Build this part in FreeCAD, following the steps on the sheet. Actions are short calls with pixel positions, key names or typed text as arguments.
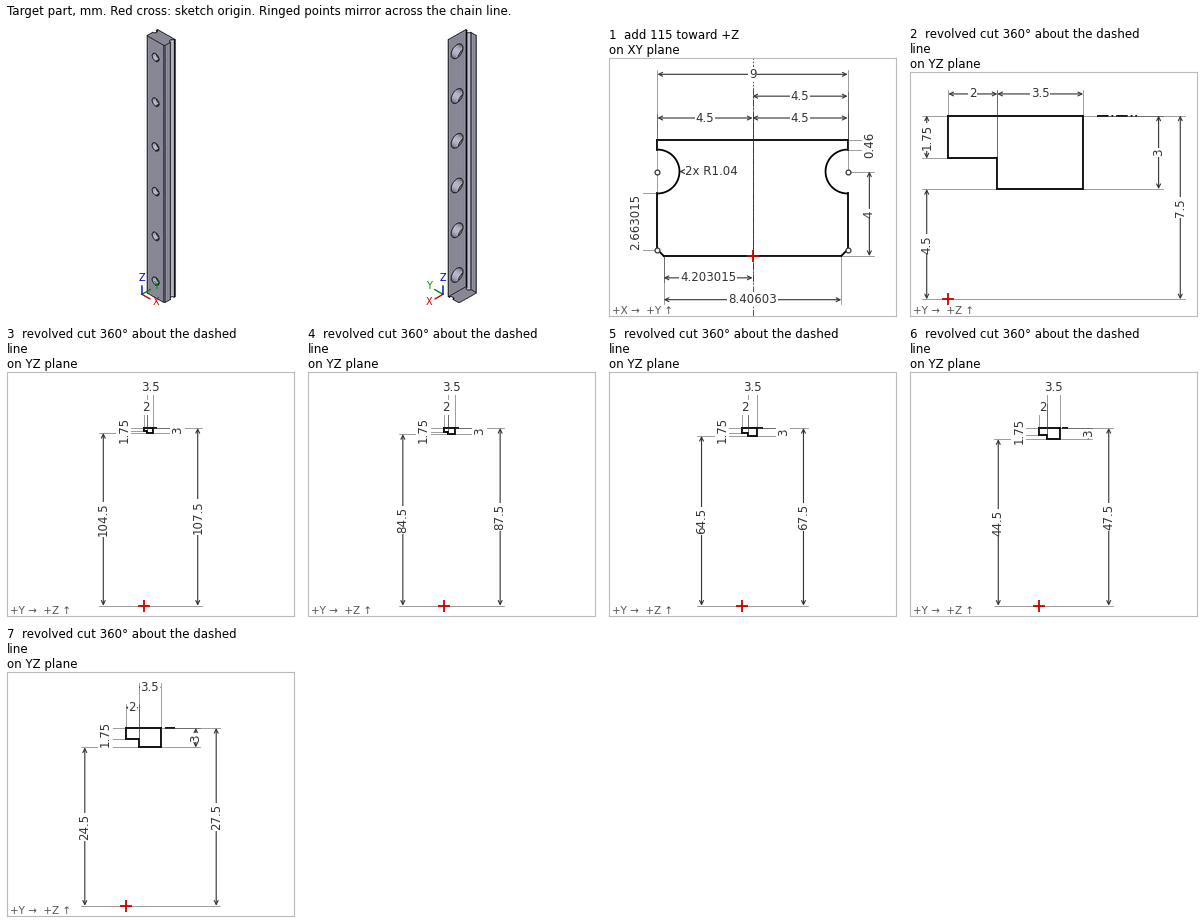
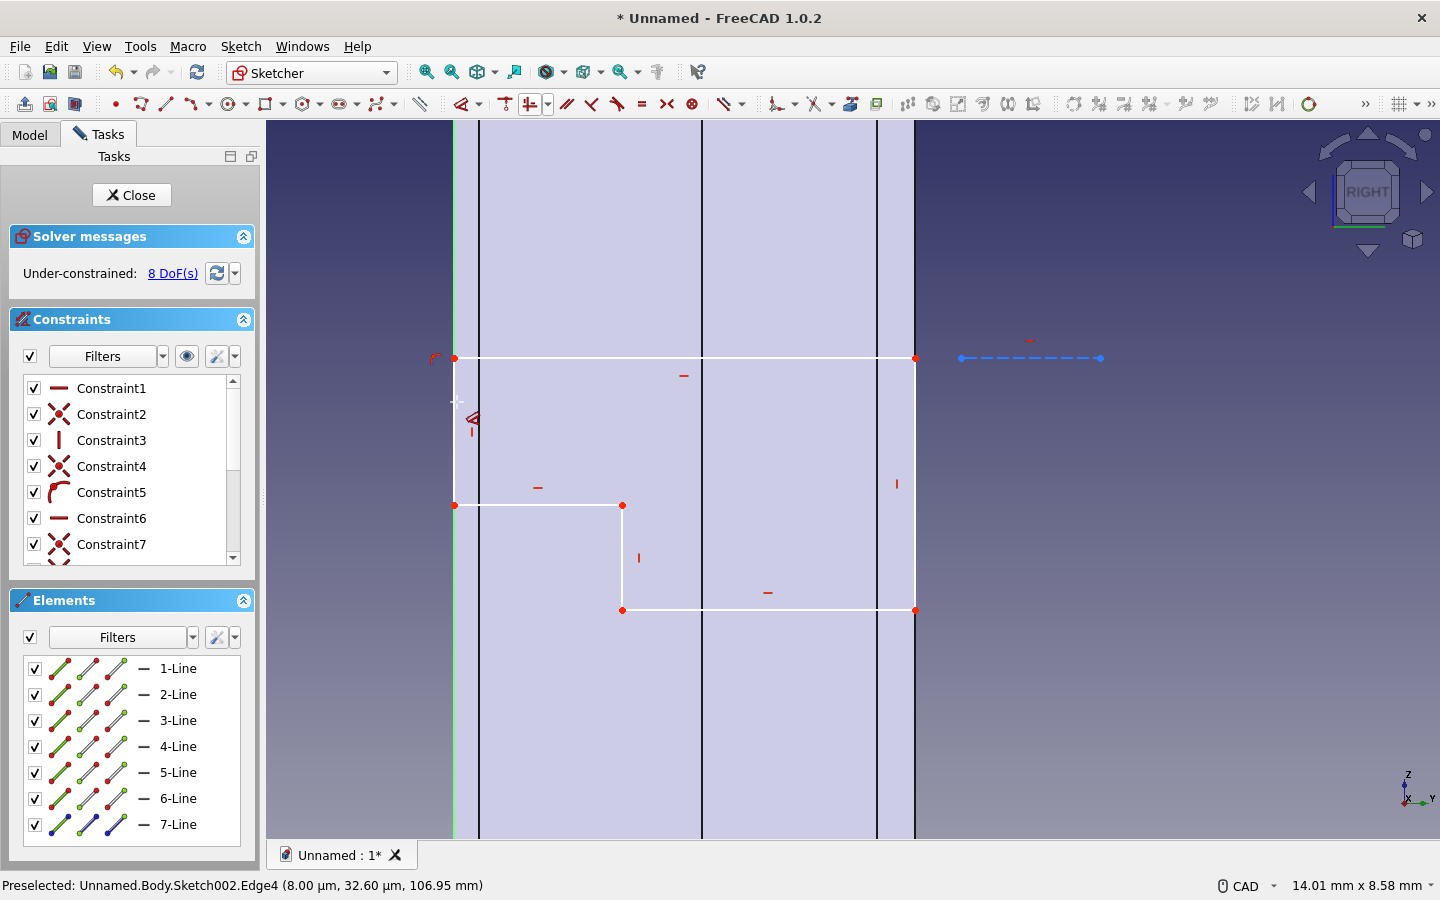
click(915, 534)
click(949, 484)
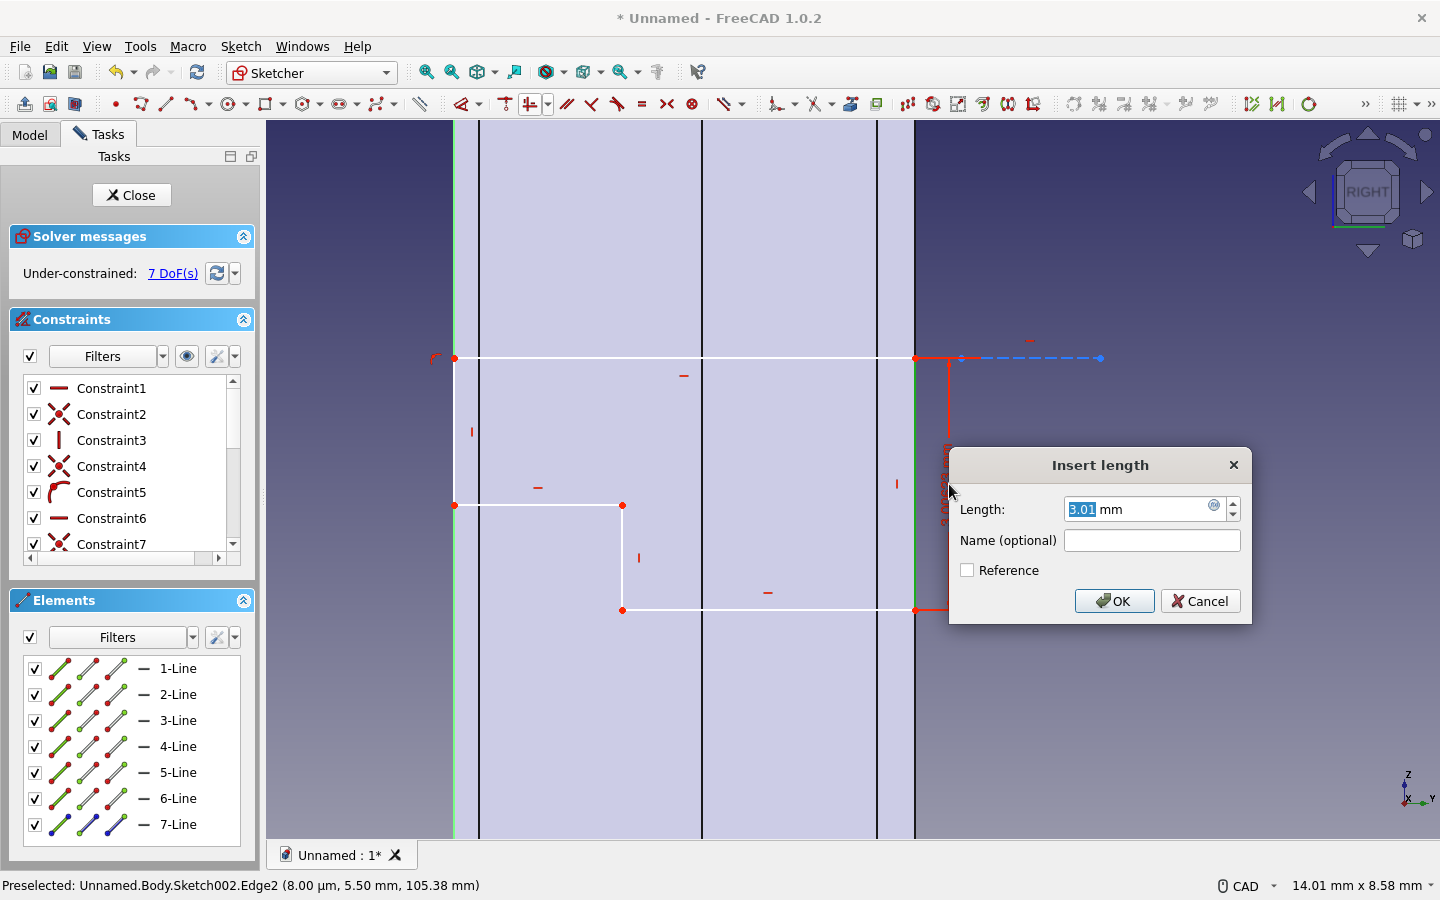
text(3)
key(Return)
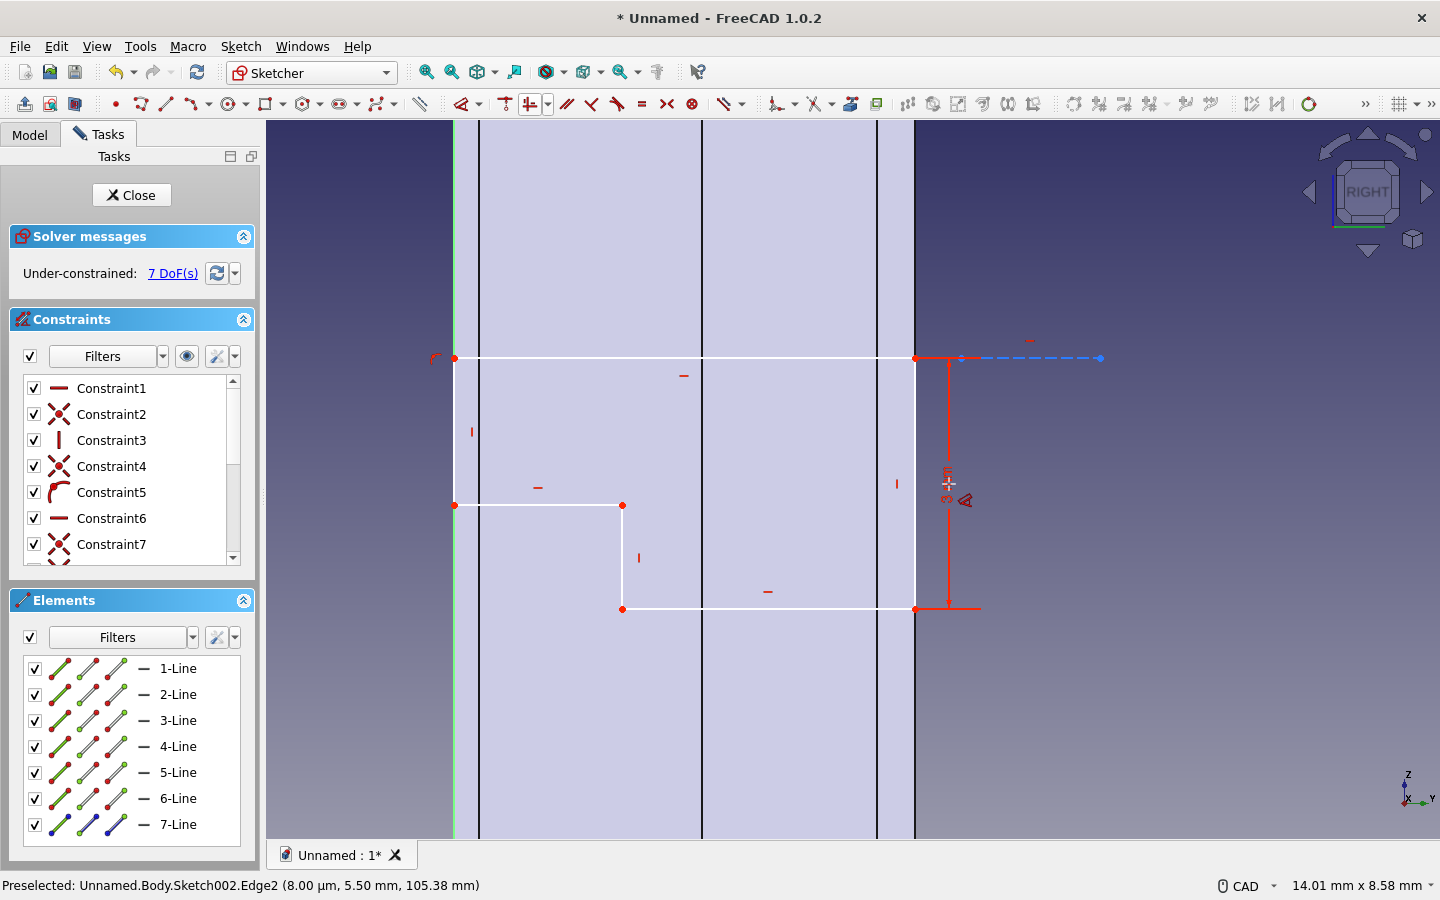
click(504, 505)
click(538, 539)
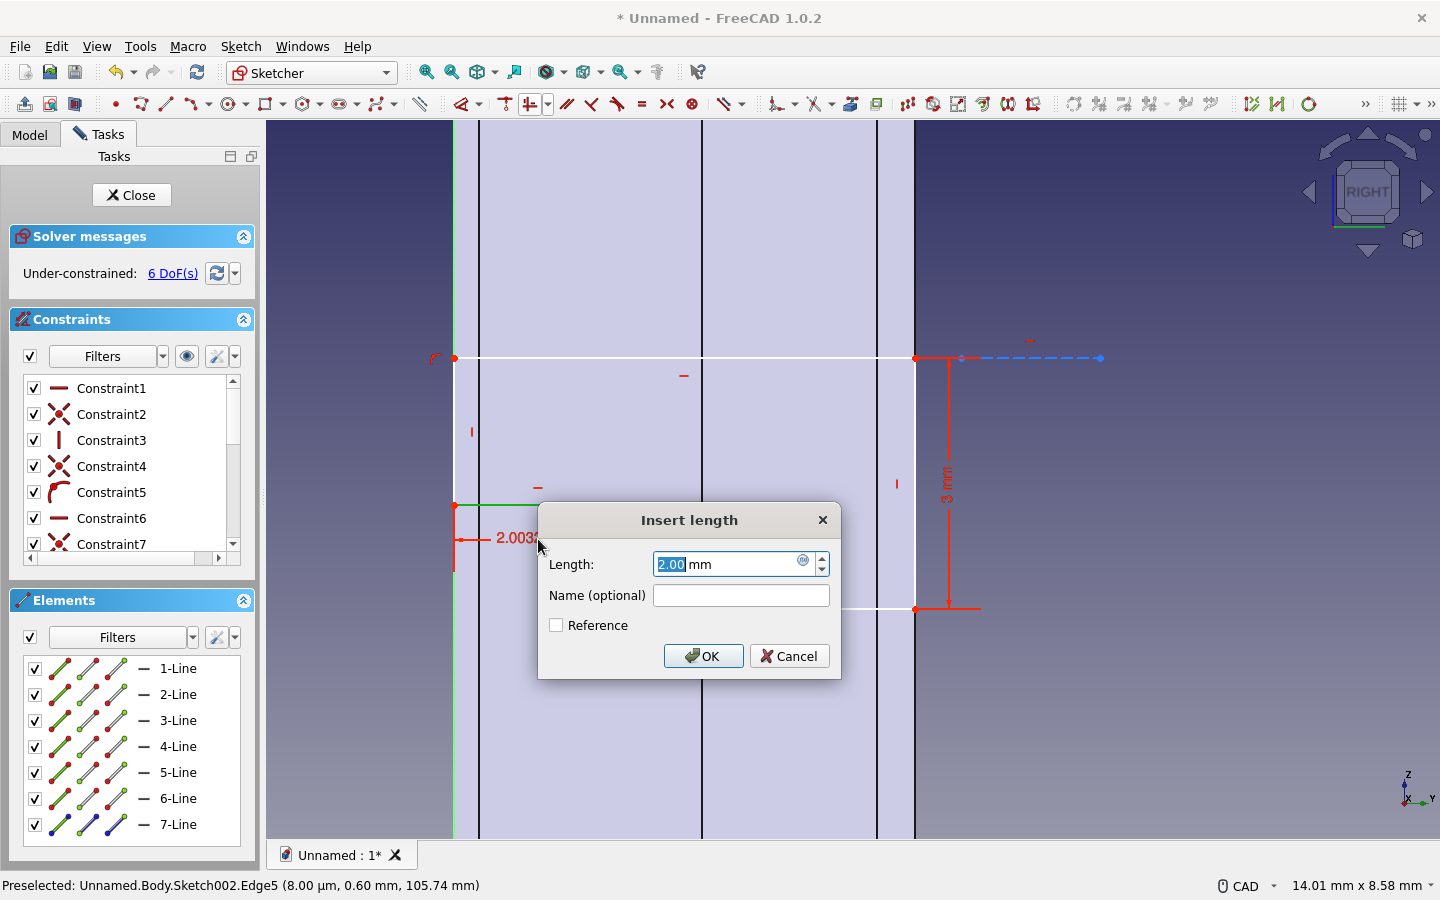
text(2)
key(Return)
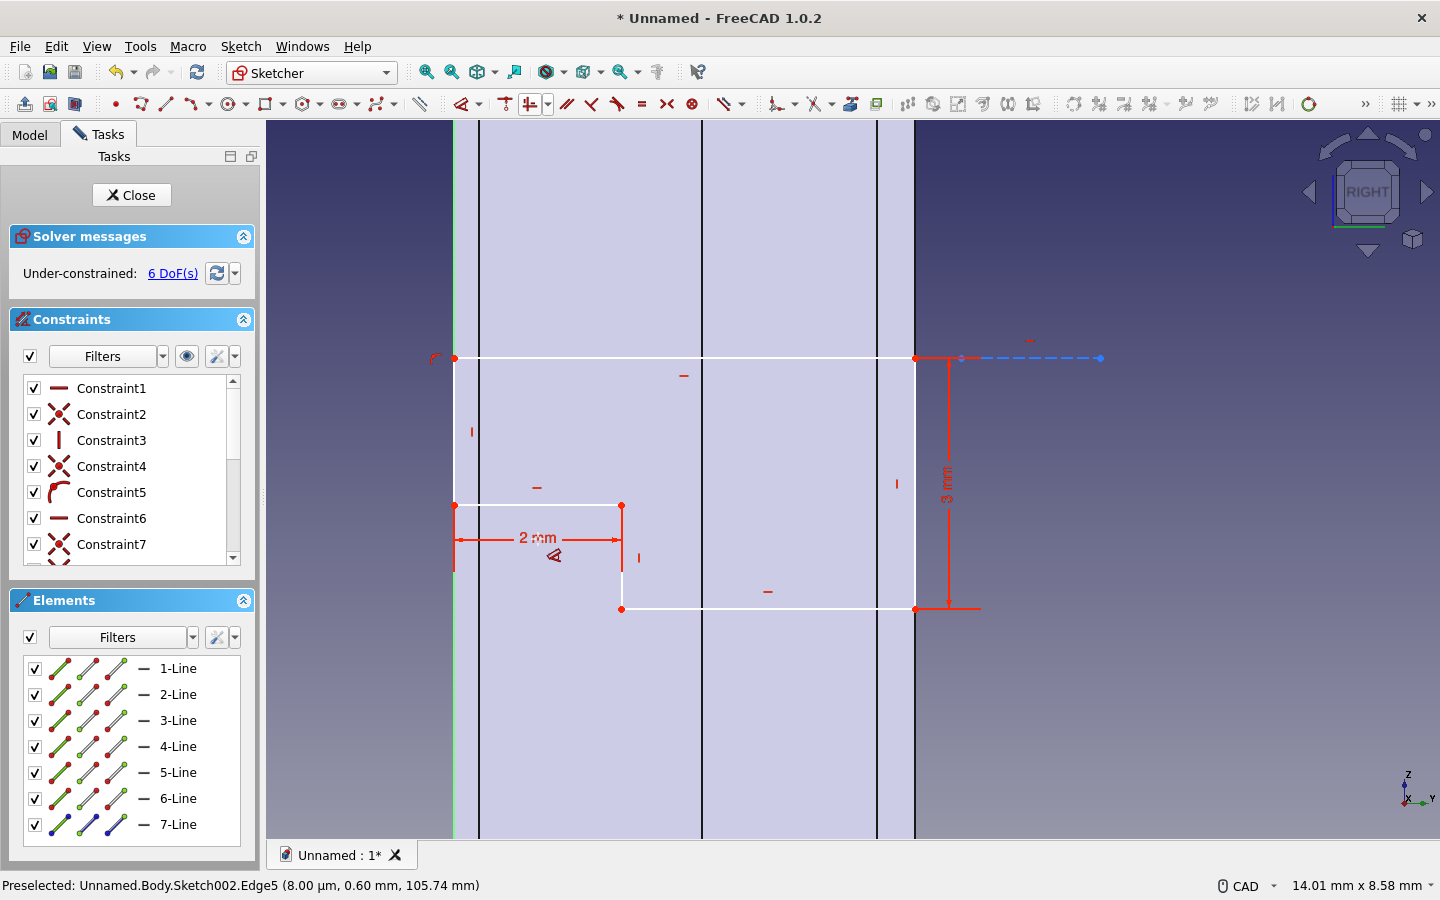
click(710, 609)
click(768, 643)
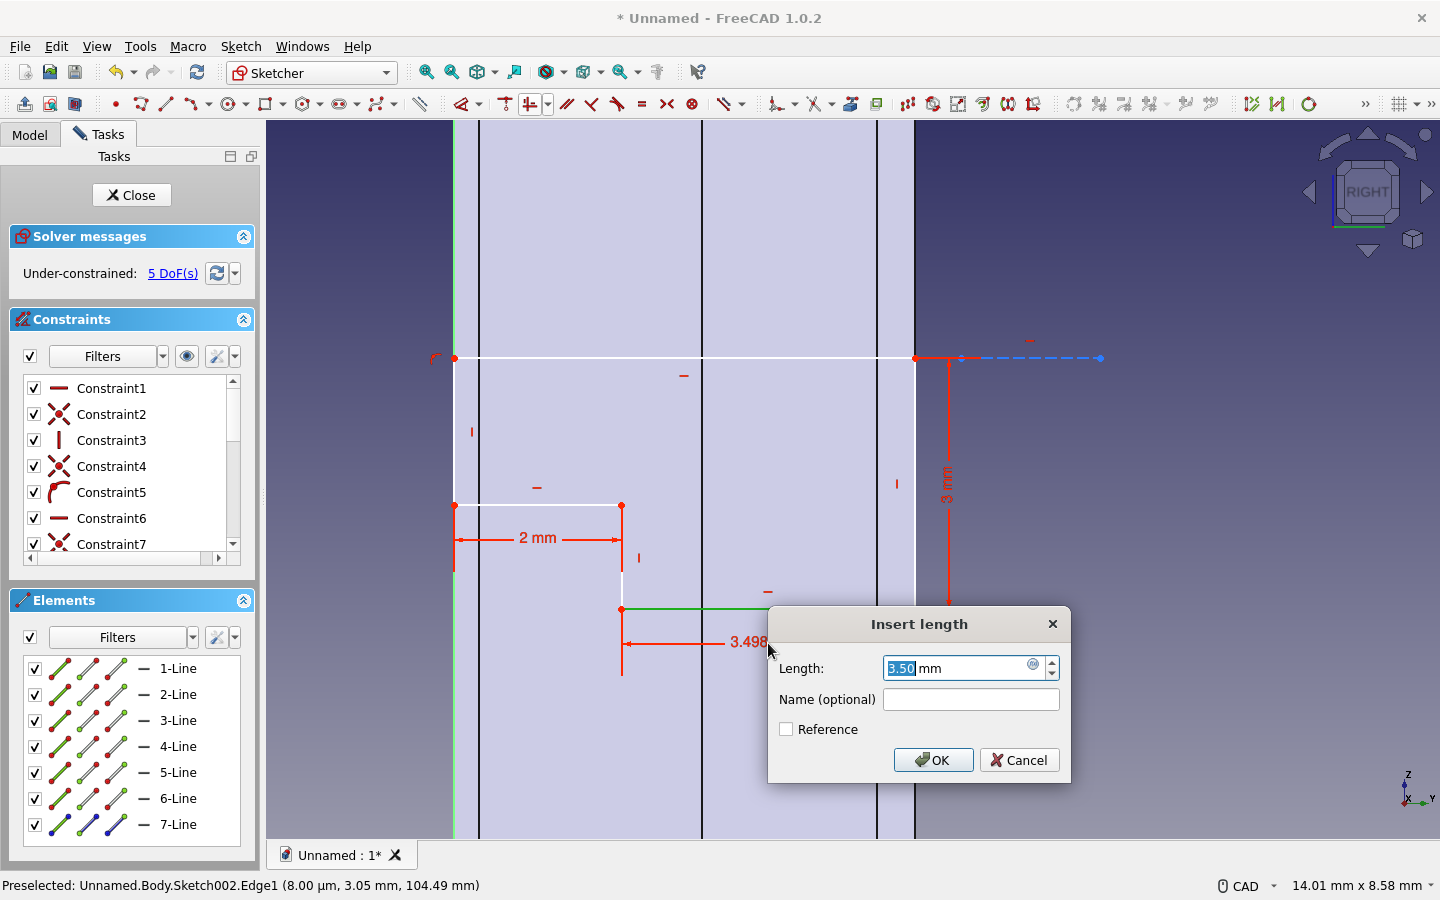
text(3.5)
key(Return)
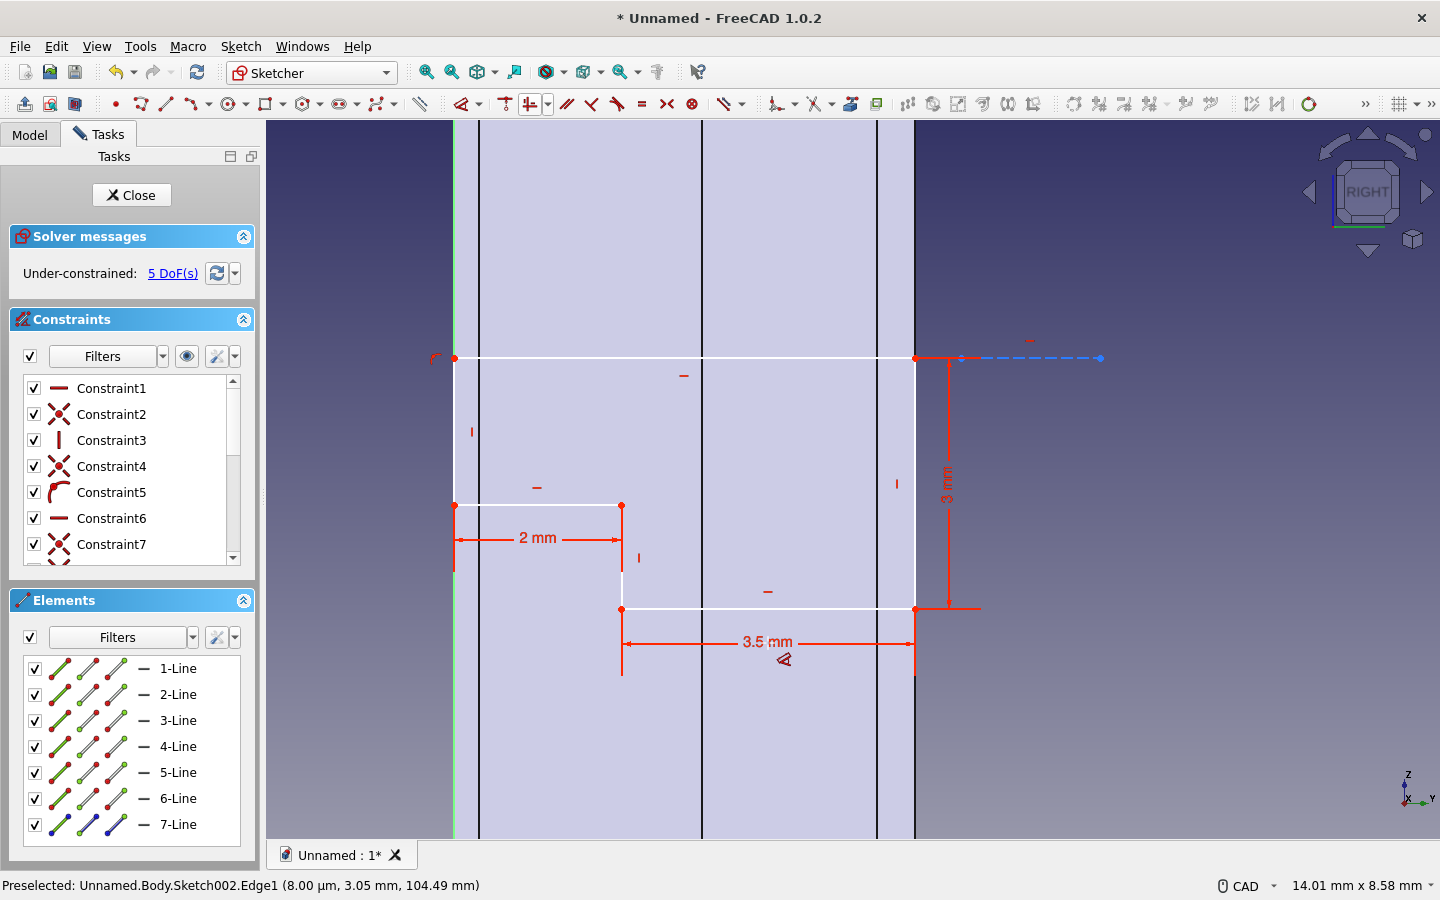
click(454, 402)
click(420, 431)